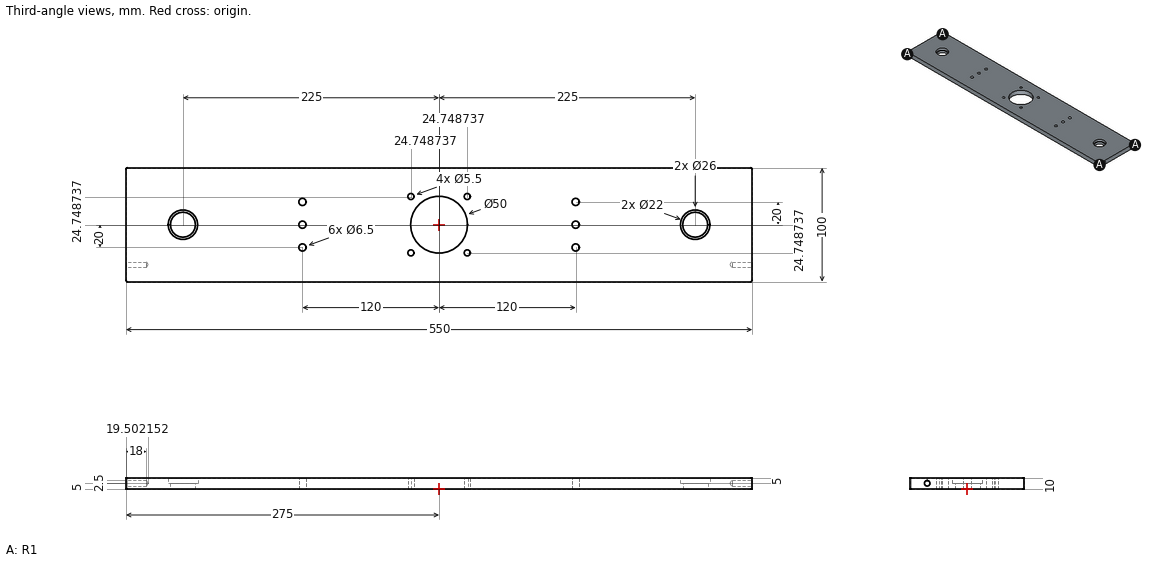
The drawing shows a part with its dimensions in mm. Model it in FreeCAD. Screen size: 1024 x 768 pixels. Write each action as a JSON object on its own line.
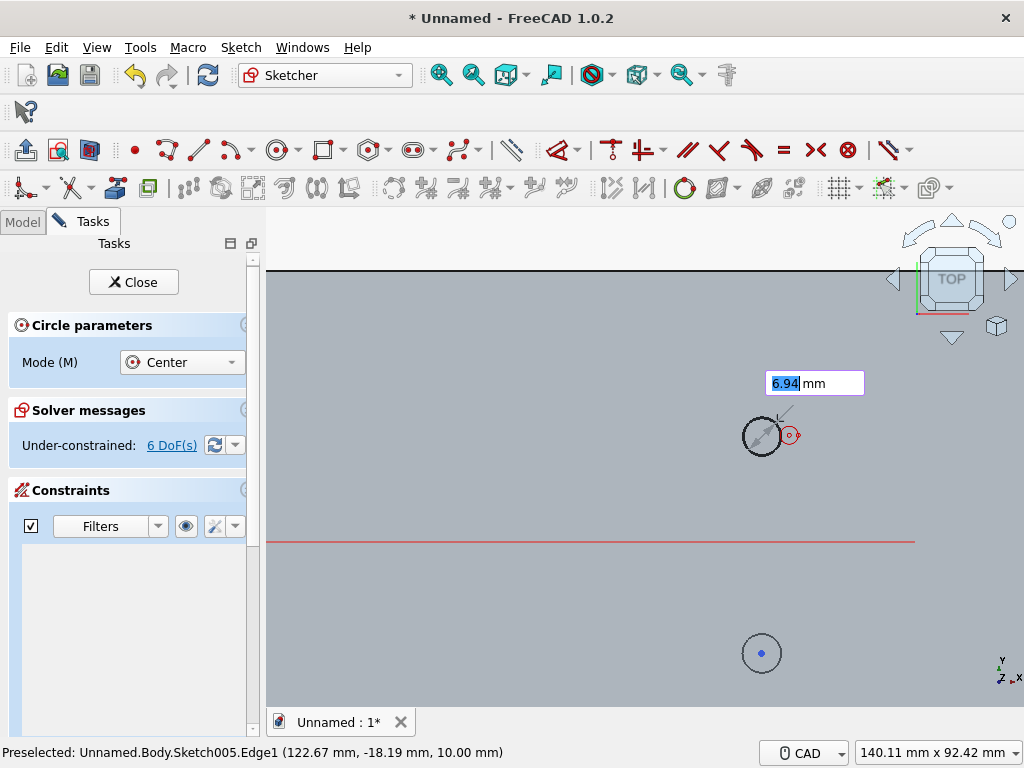
{"action": "left_click", "coordinate": [774, 421]}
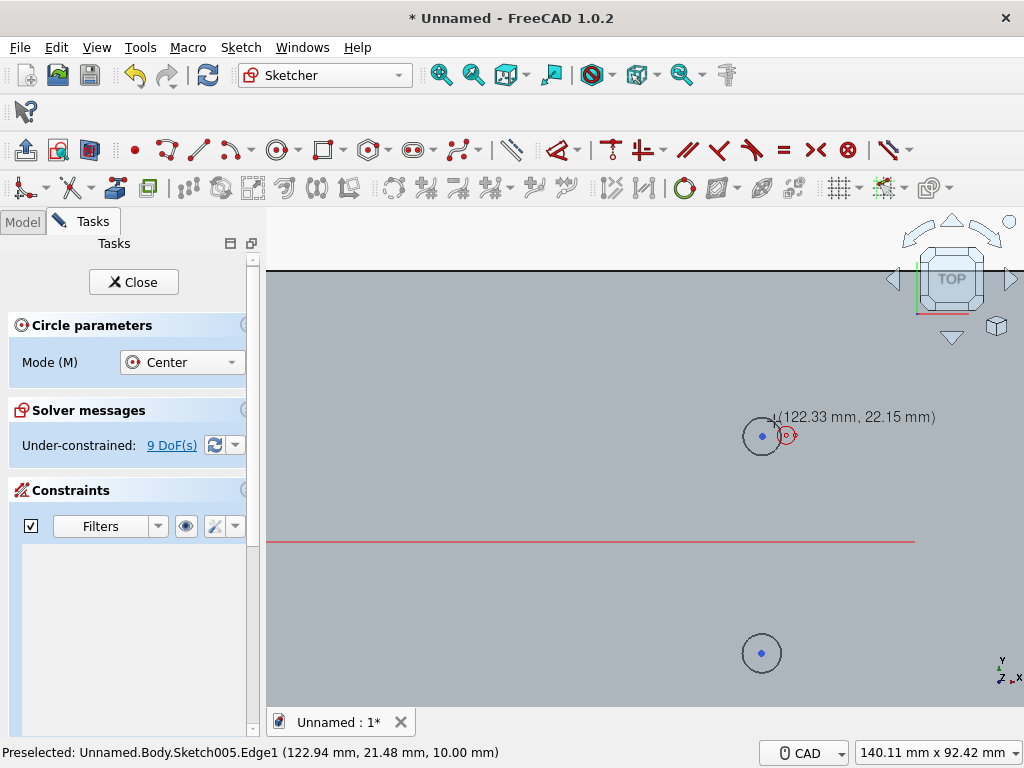
{"action": "scroll", "coordinate": [777, 420], "scroll_direction": "down", "scroll_amount": 6}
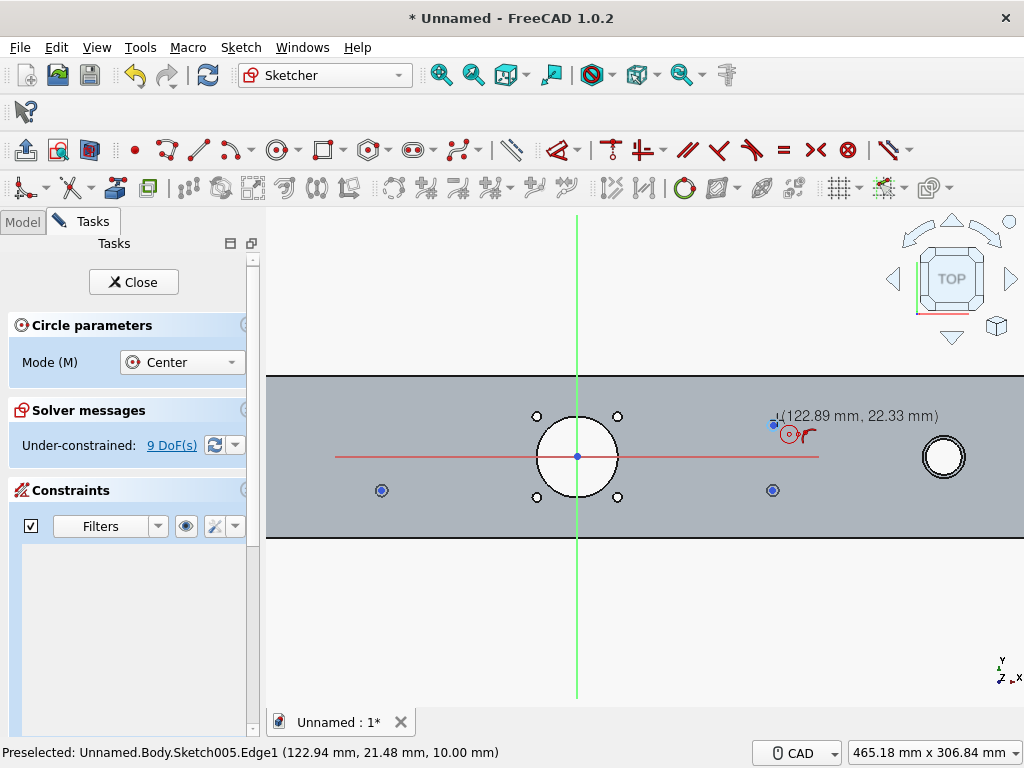
{"action": "scroll", "coordinate": [382, 424], "scroll_direction": "up", "scroll_amount": 8}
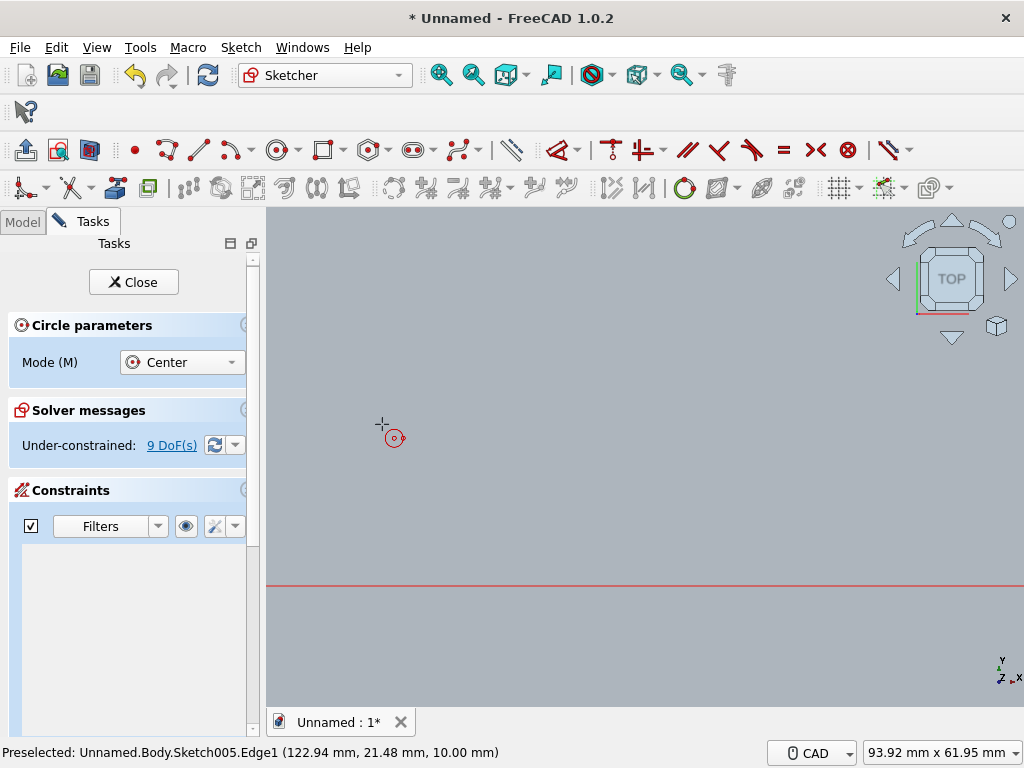
{"action": "scroll", "coordinate": [381, 424], "scroll_direction": "down", "scroll_amount": 8}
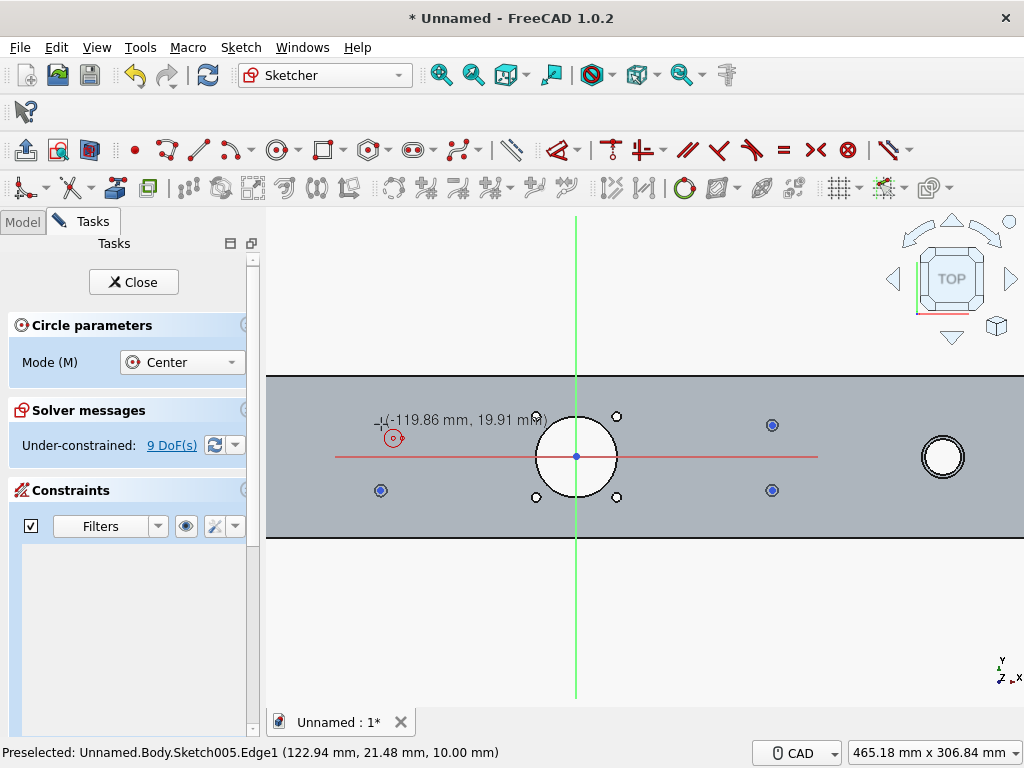
{"action": "left_click", "coordinate": [381, 424]}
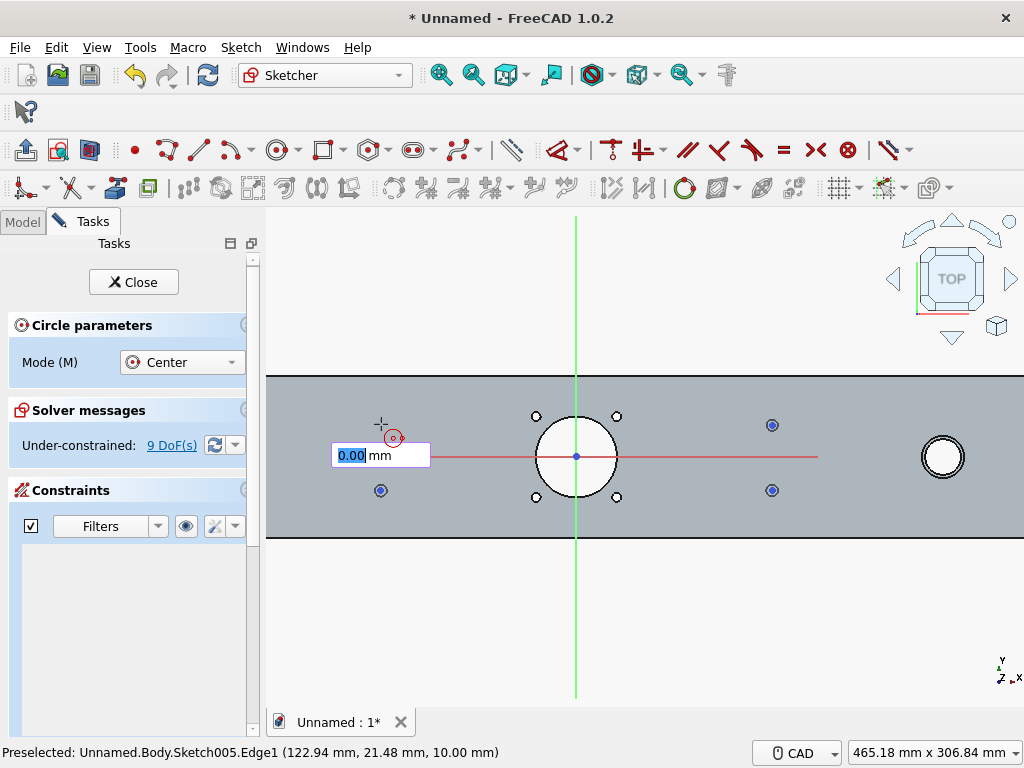
{"action": "scroll", "coordinate": [385, 421], "scroll_direction": "up", "scroll_amount": 6}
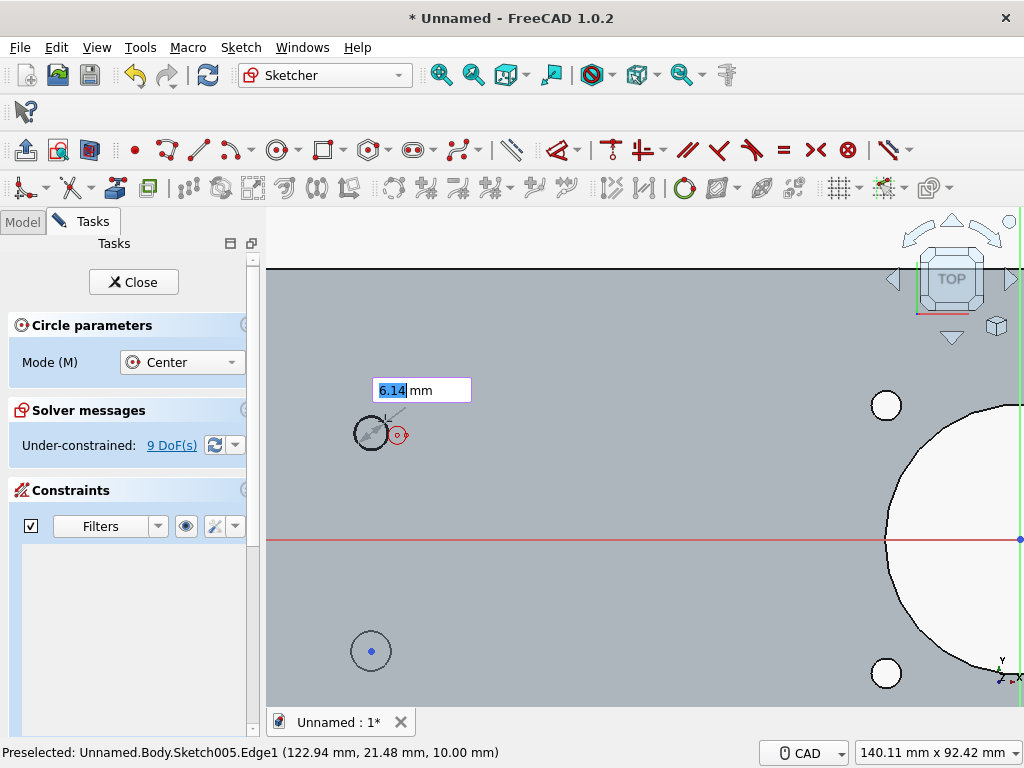
{"action": "left_click", "coordinate": [383, 419]}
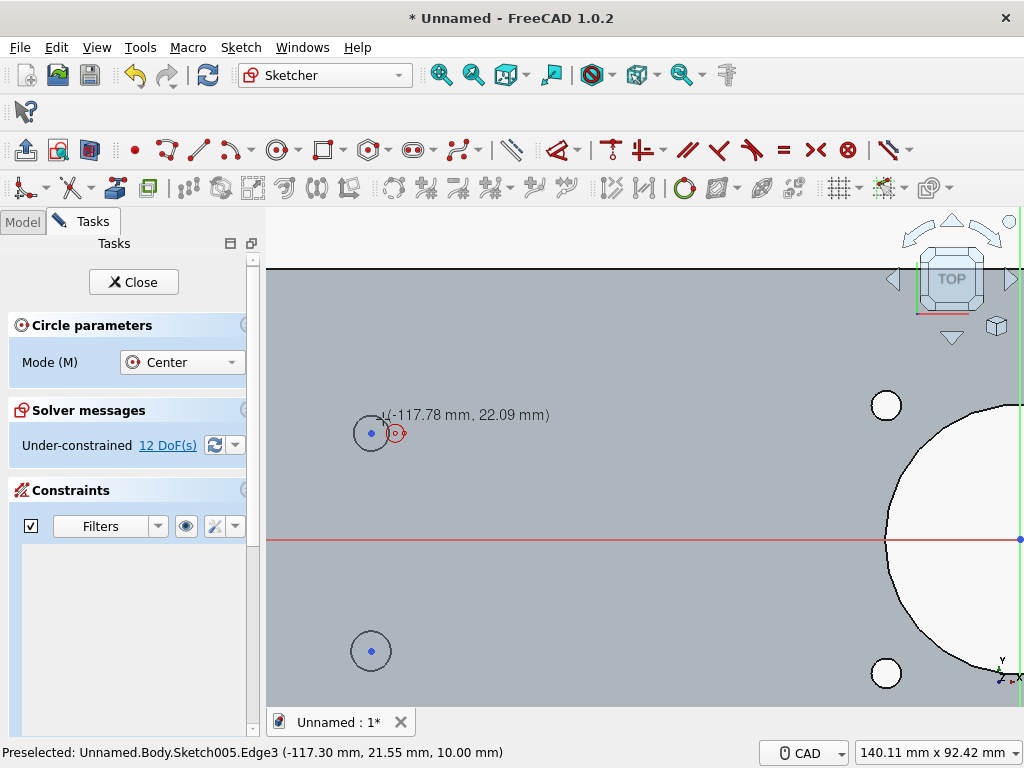
{"action": "scroll", "coordinate": [371, 540], "scroll_direction": "up", "scroll_amount": 2}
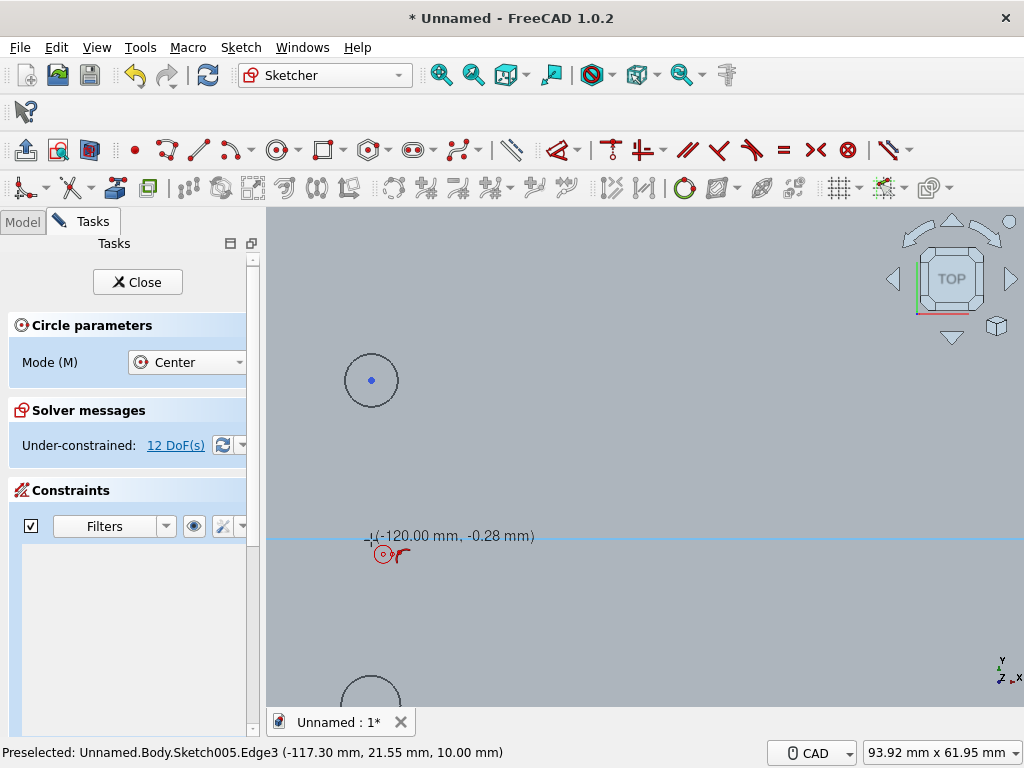
{"action": "scroll", "coordinate": [384, 436], "scroll_direction": "down", "scroll_amount": 8}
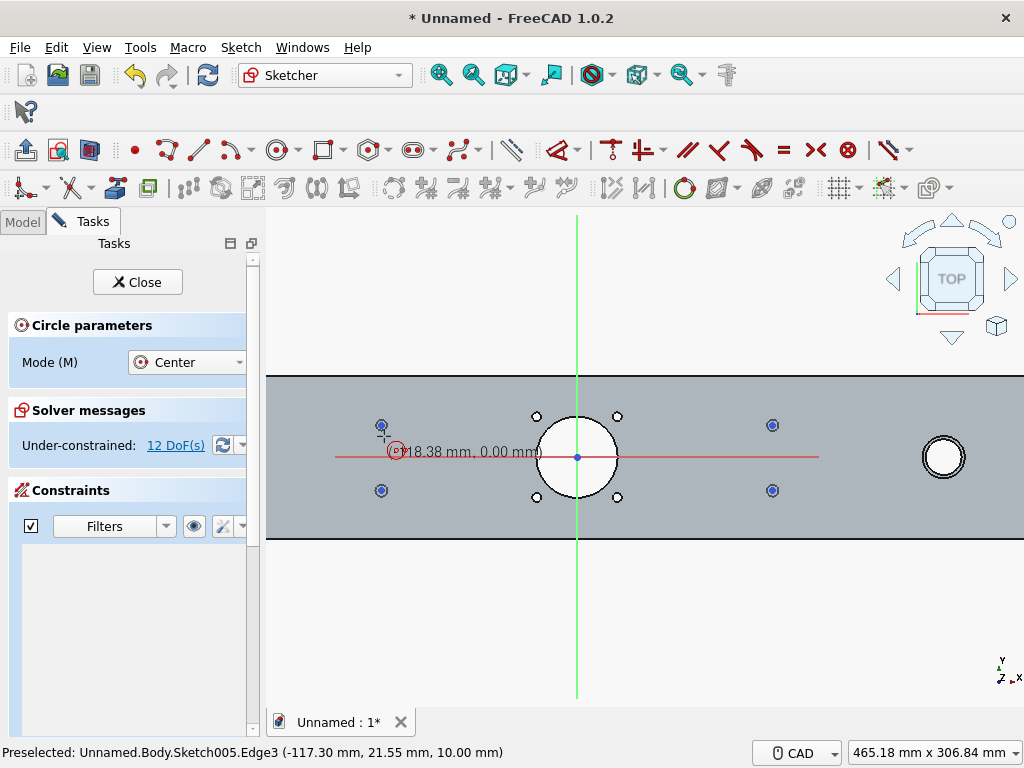
{"action": "left_click", "coordinate": [381, 457]}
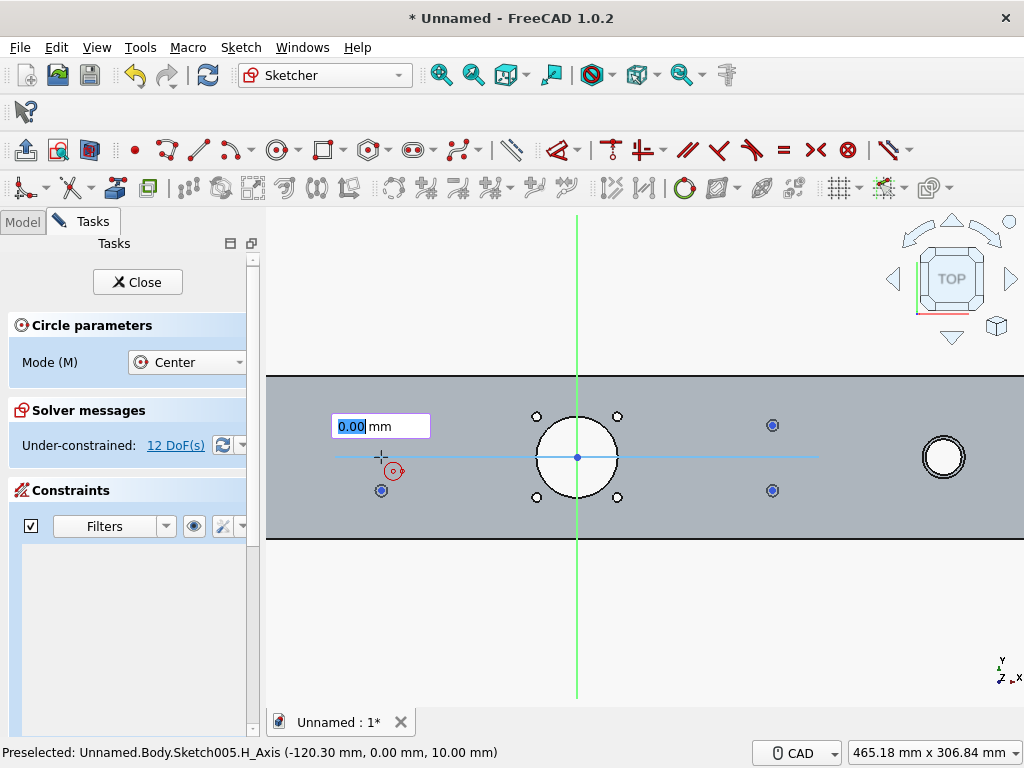
{"action": "scroll", "coordinate": [380, 462], "scroll_direction": "up", "scroll_amount": 6}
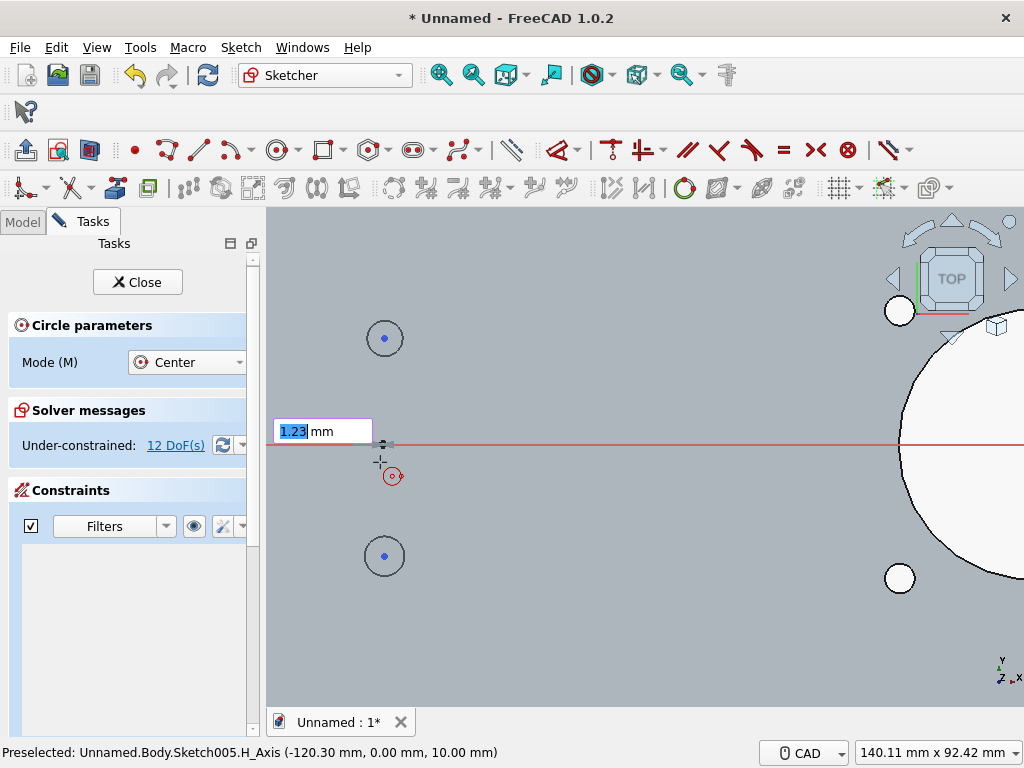
{"action": "left_click", "coordinate": [379, 461]}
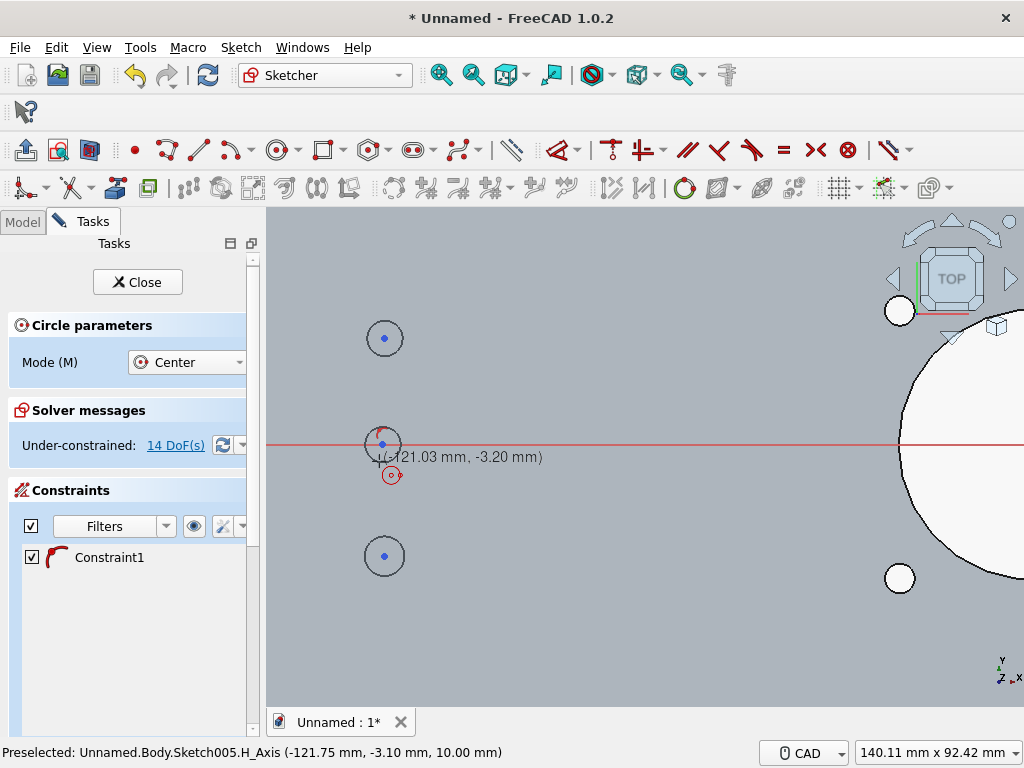
{"action": "scroll", "coordinate": [379, 462], "scroll_direction": "down", "scroll_amount": 6}